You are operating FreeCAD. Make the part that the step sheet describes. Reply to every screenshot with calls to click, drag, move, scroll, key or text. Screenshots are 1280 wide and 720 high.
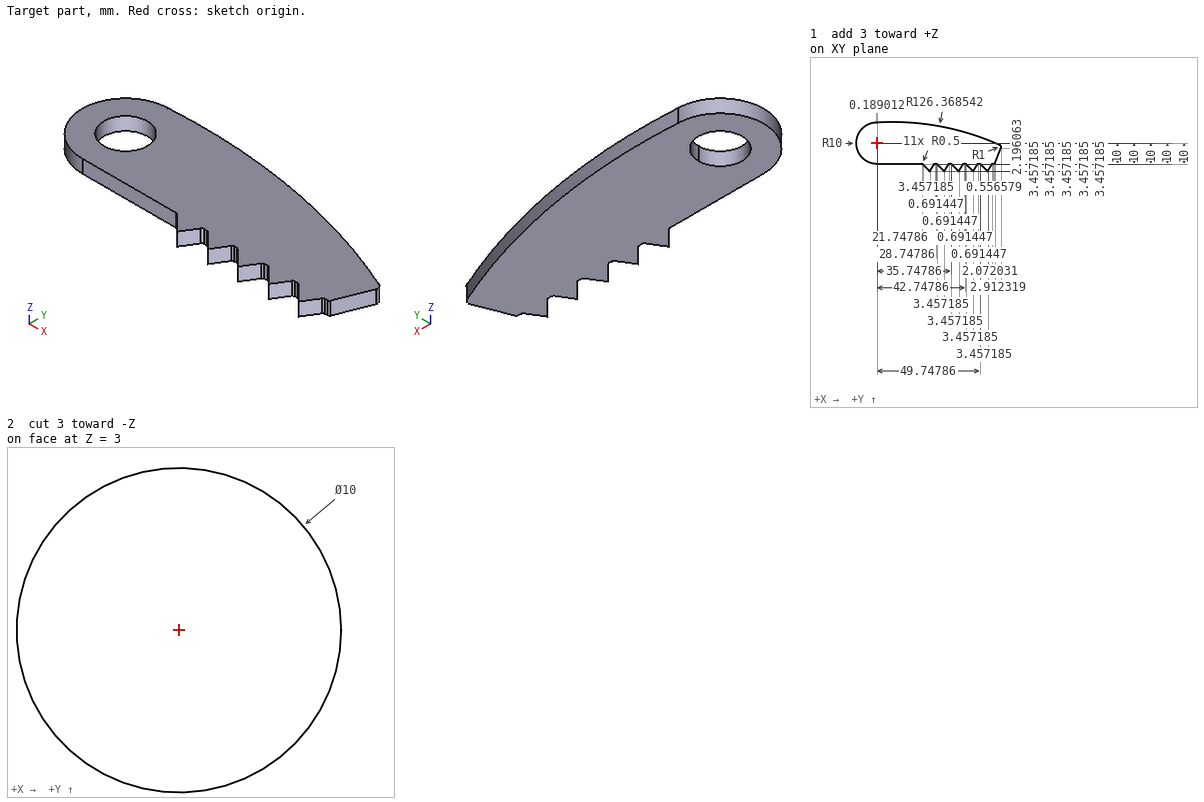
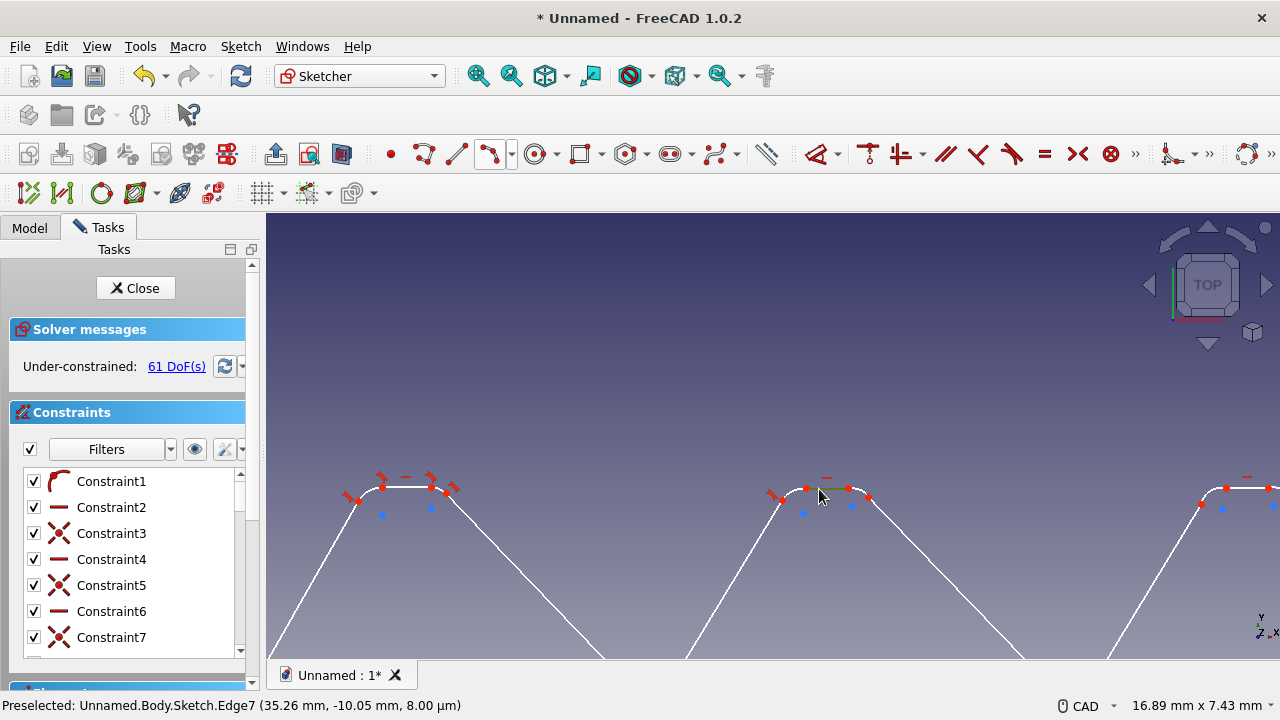
click(793, 491)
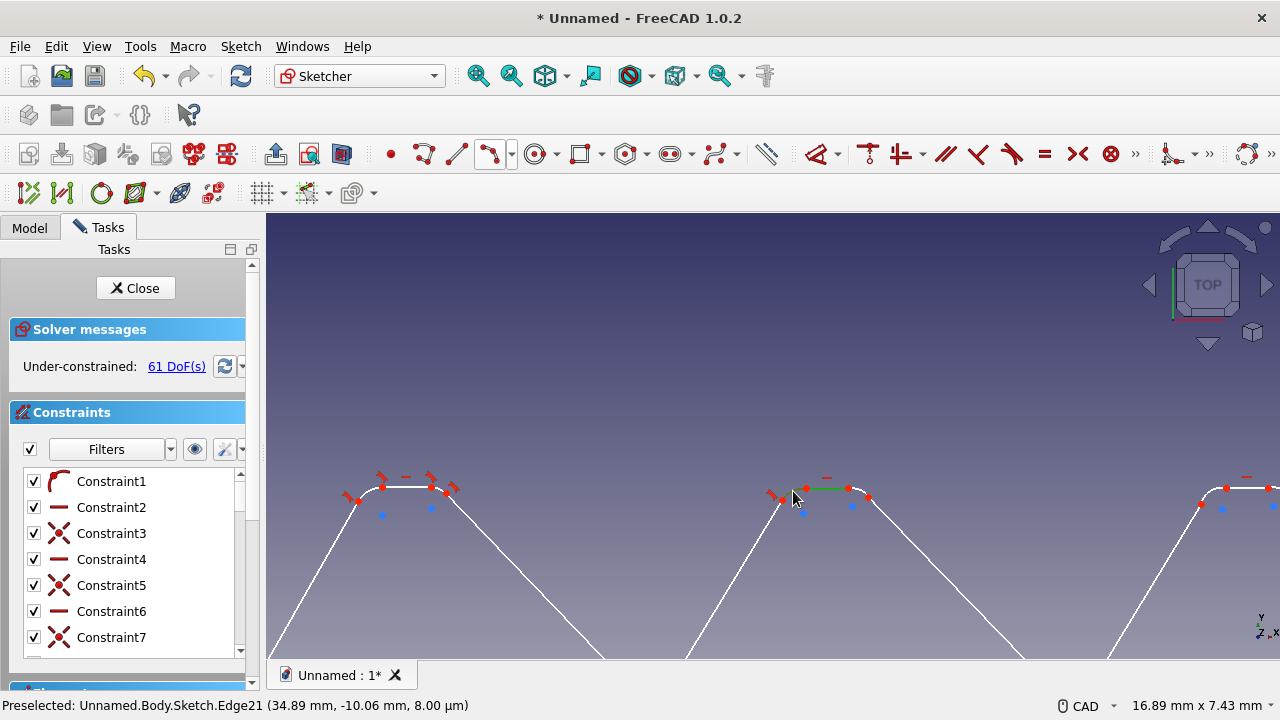
click(1012, 154)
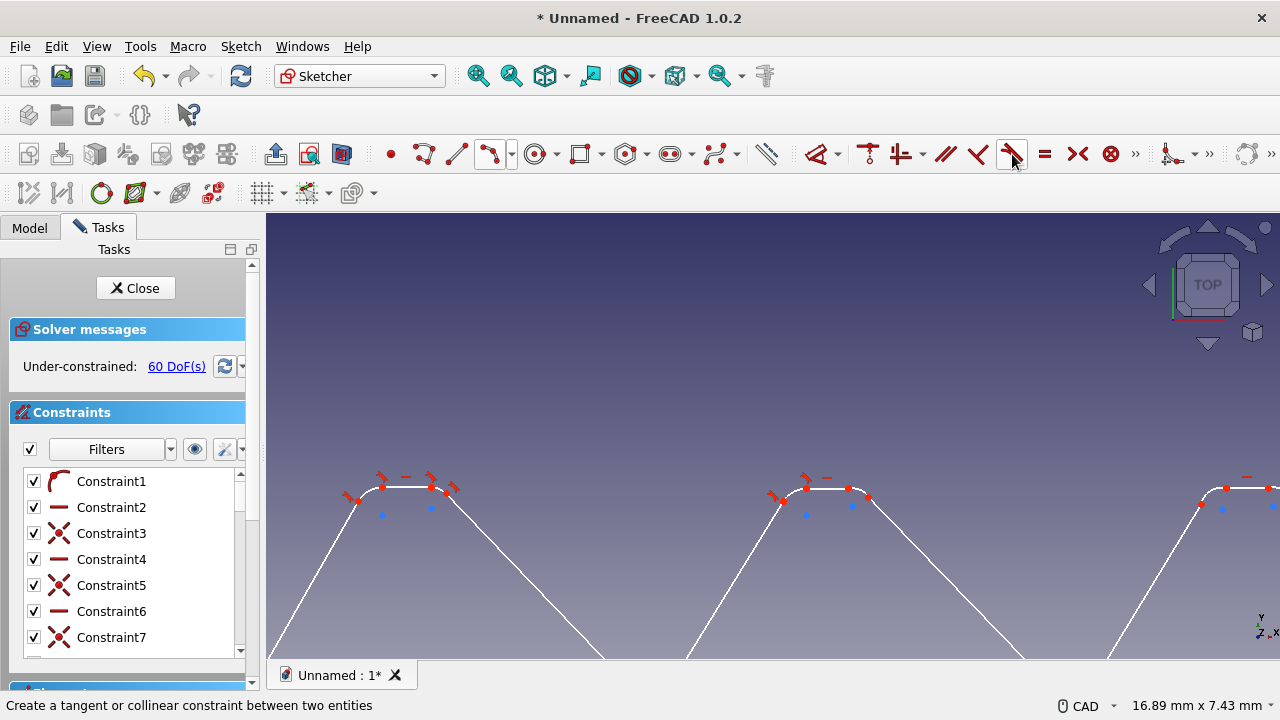
click(819, 489)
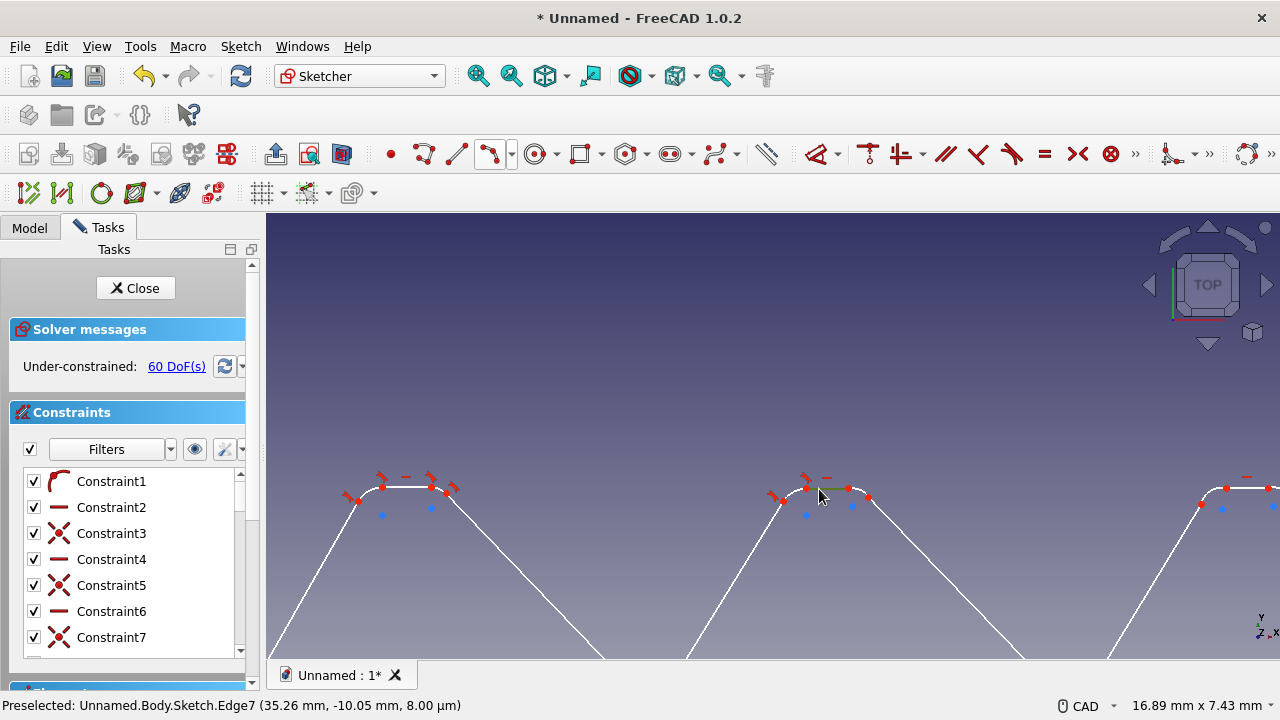
click(860, 490)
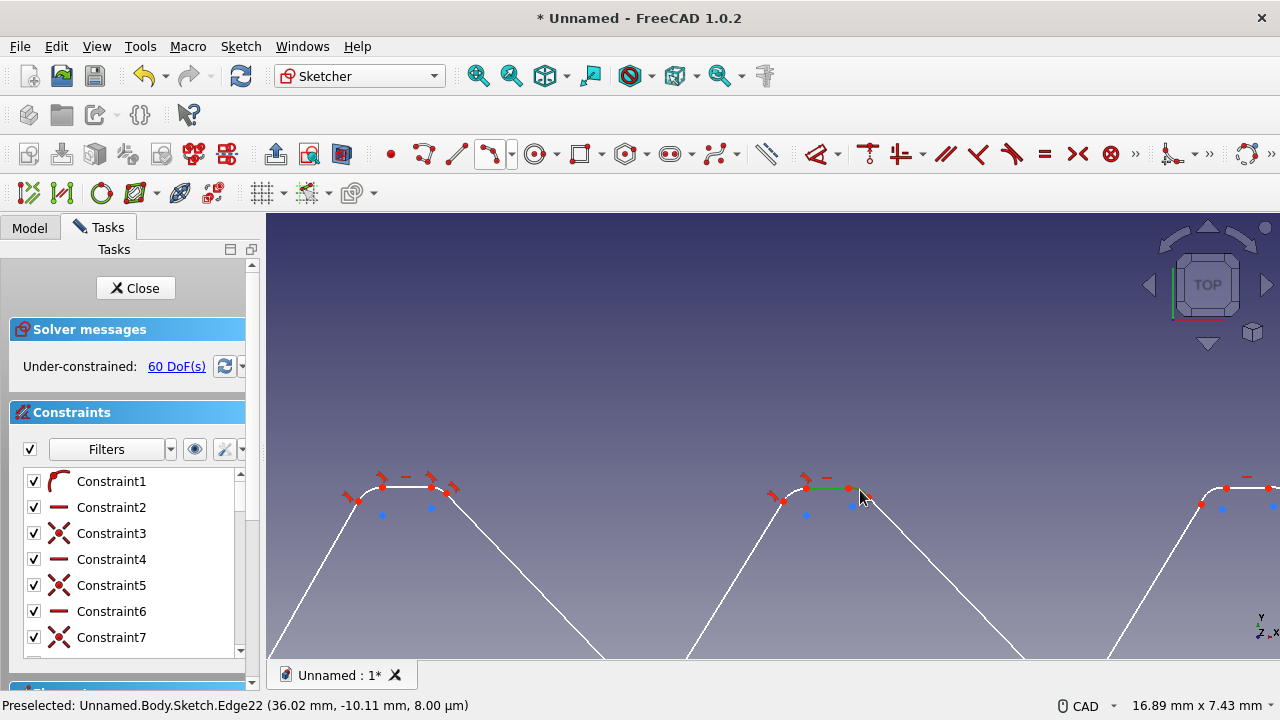
click(1012, 154)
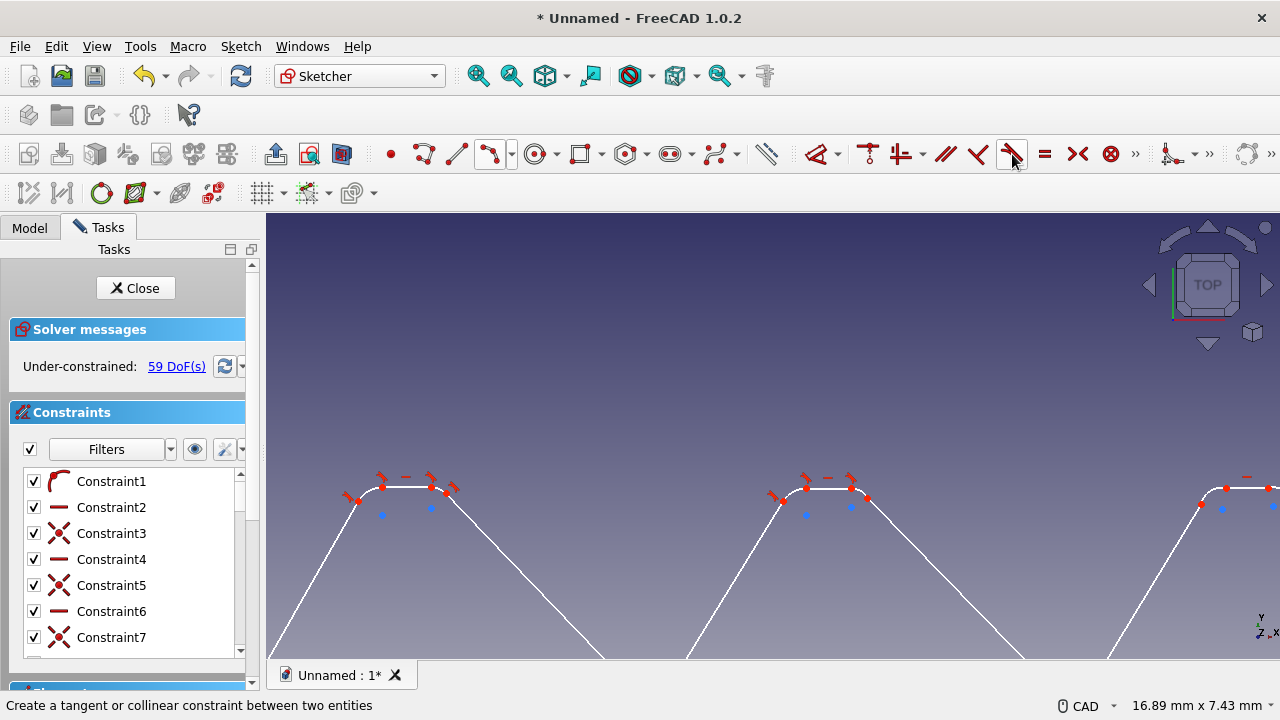
scroll(783, 505, down, 10)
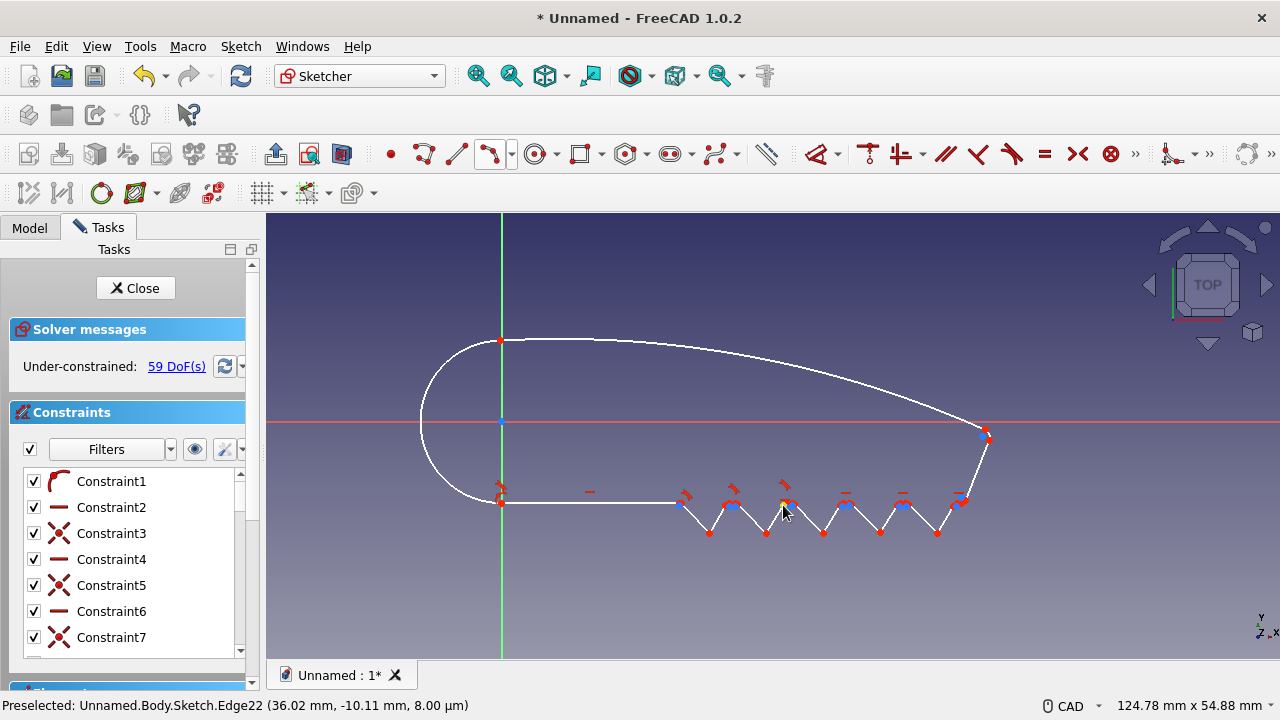
click(803, 513)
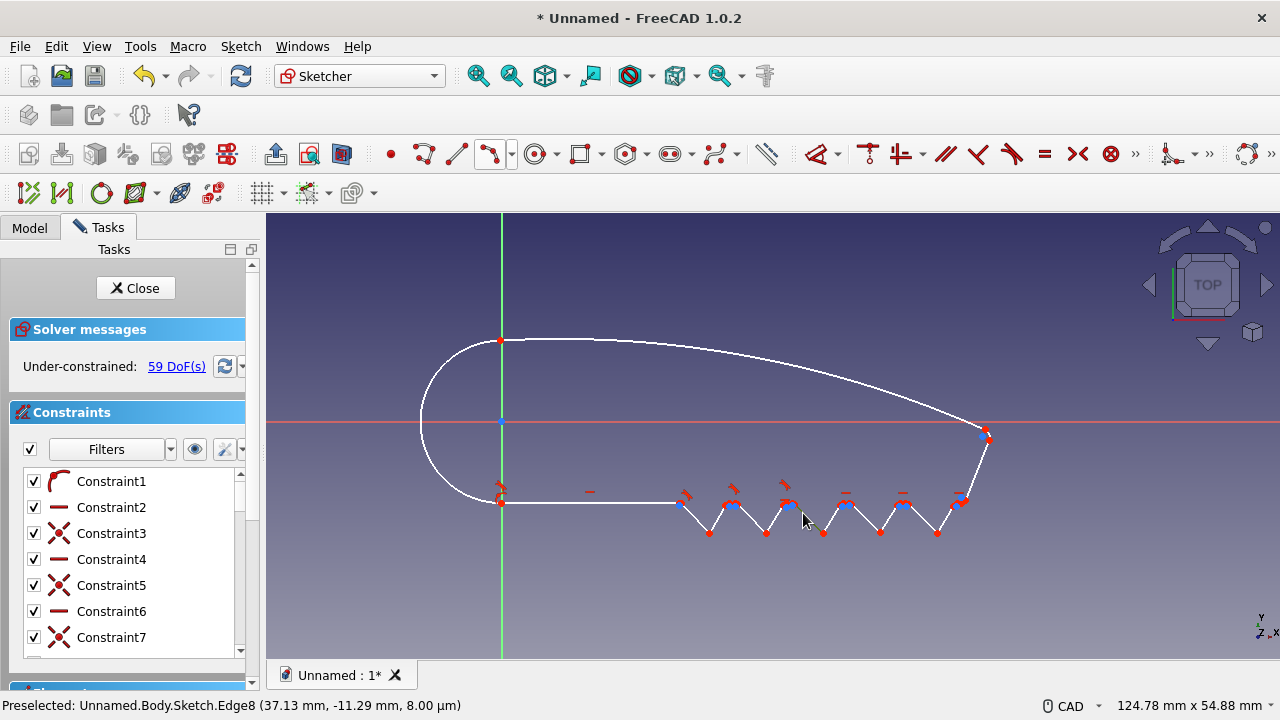
scroll(794, 504, up, 12)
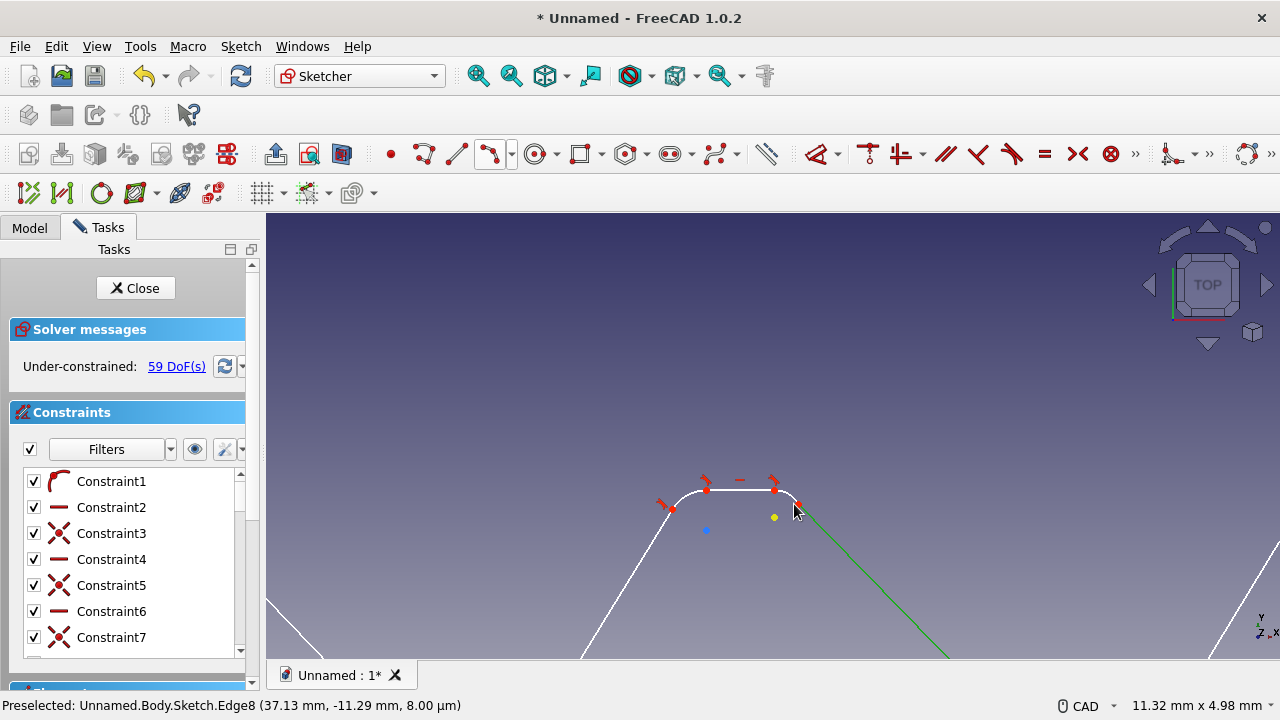
click(789, 494)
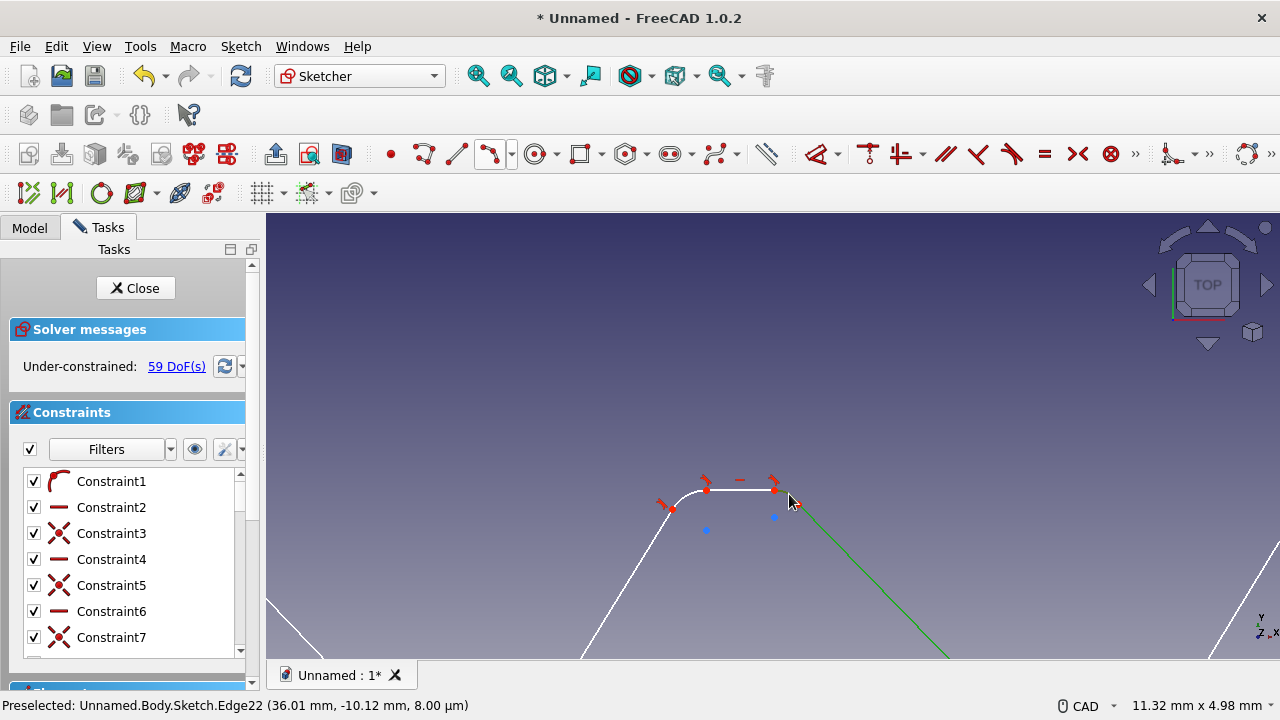
key(t)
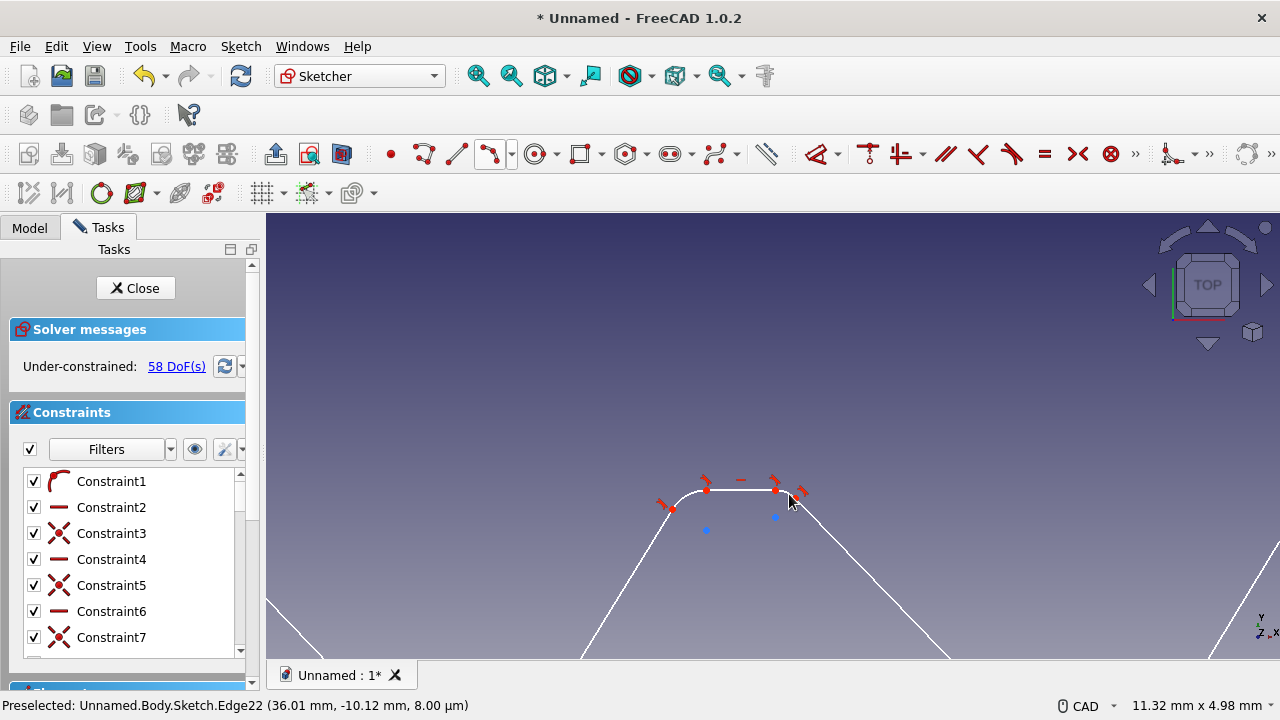
scroll(794, 504, down, 12)